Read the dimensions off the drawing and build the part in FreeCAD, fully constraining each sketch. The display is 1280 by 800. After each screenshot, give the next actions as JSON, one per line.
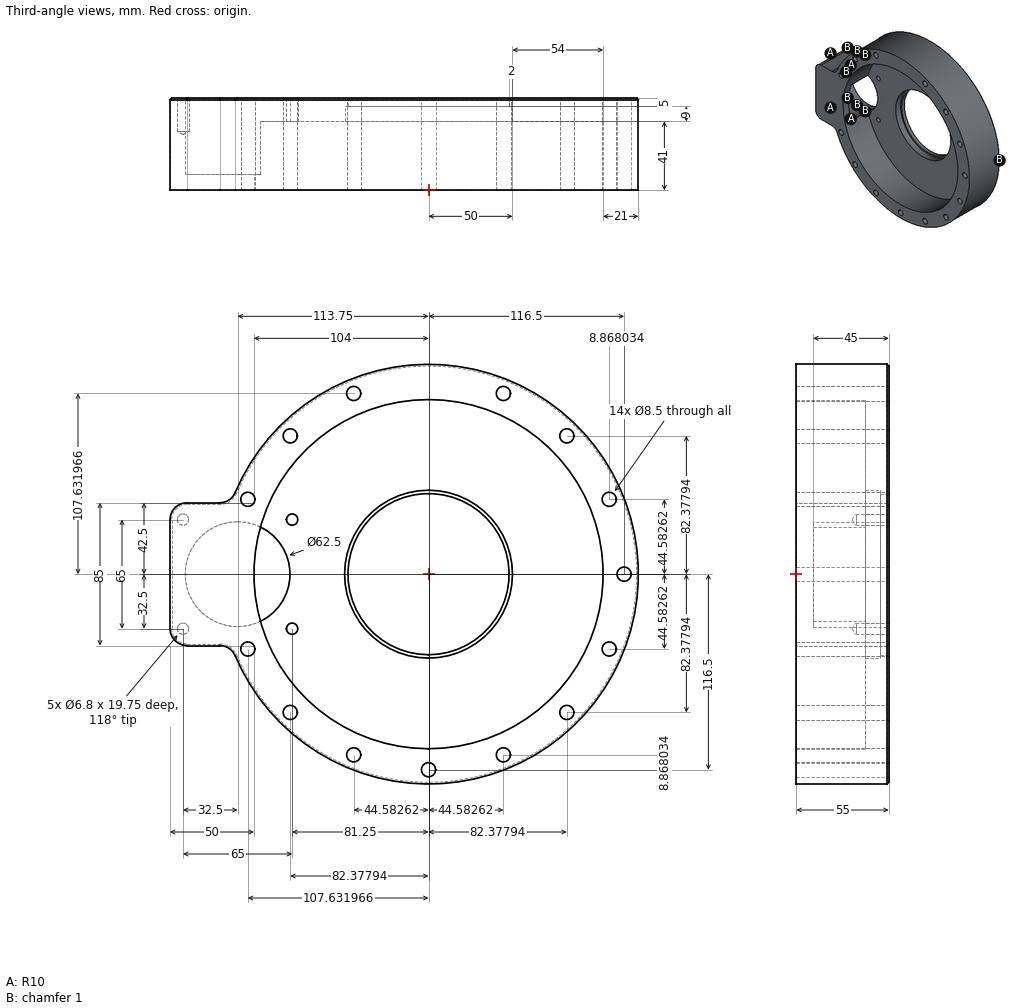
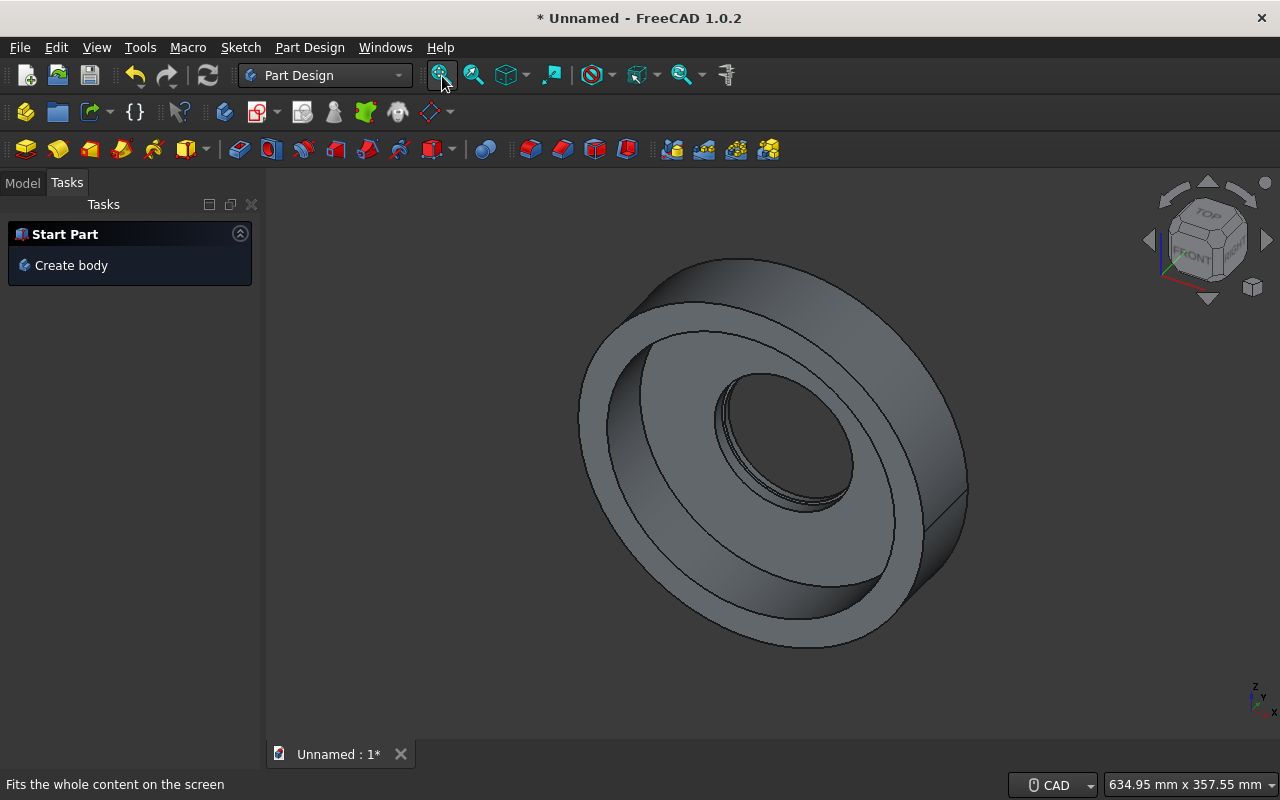
{"action": "key", "text": "4"}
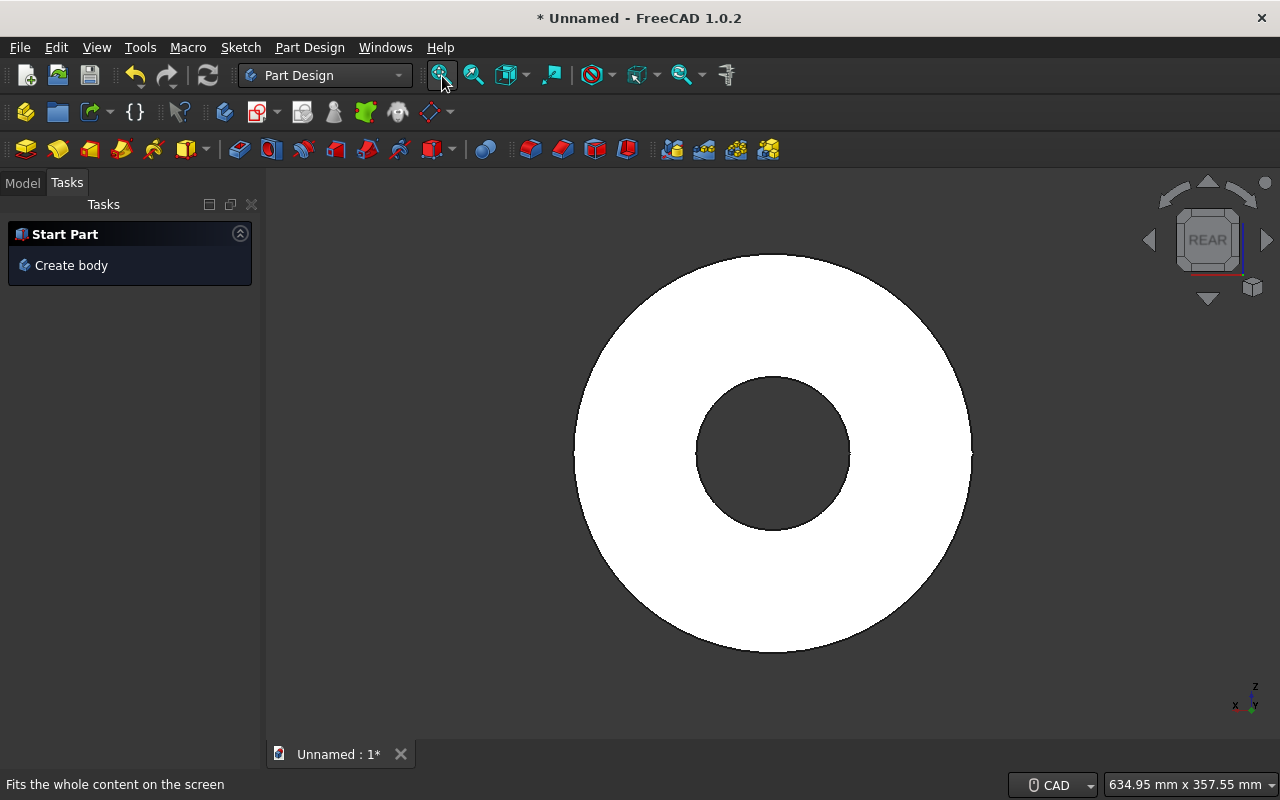
{"action": "left_click", "coordinate": [716, 567]}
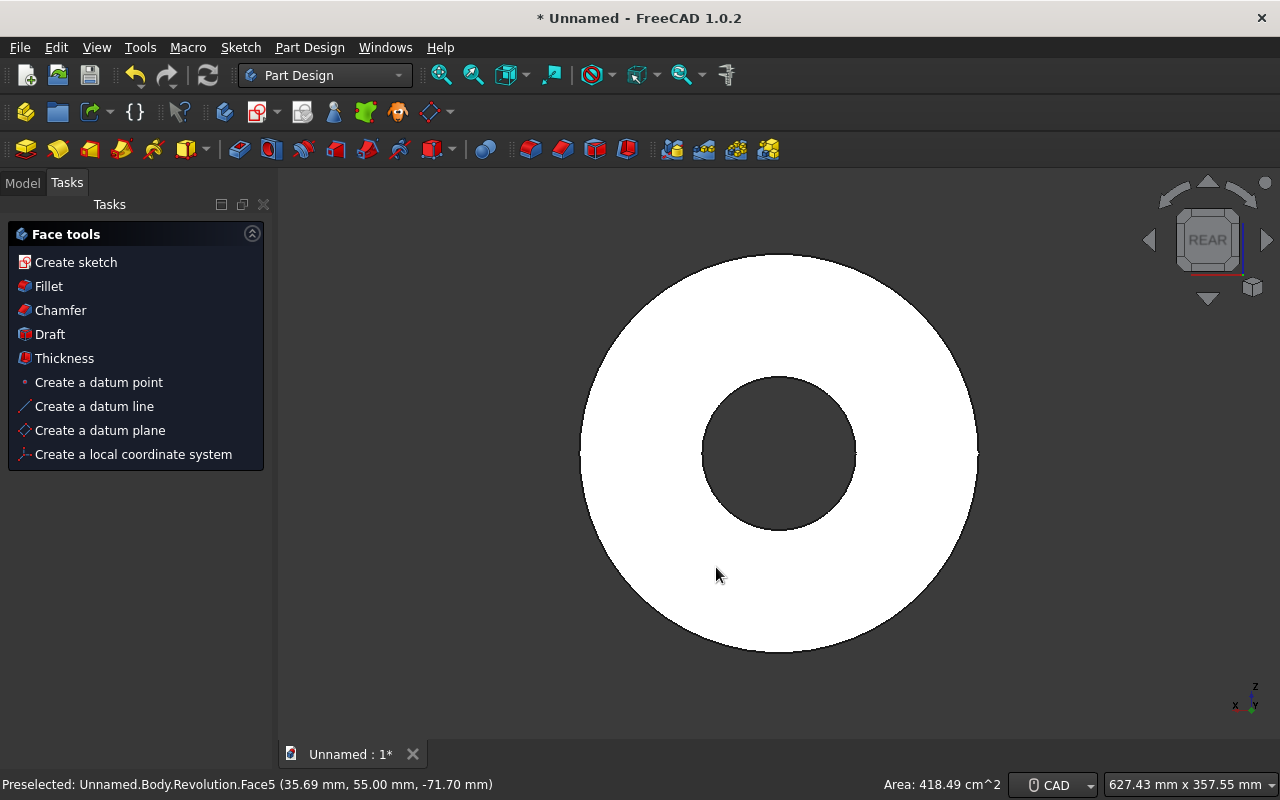
{"action": "left_click", "coordinate": [258, 112]}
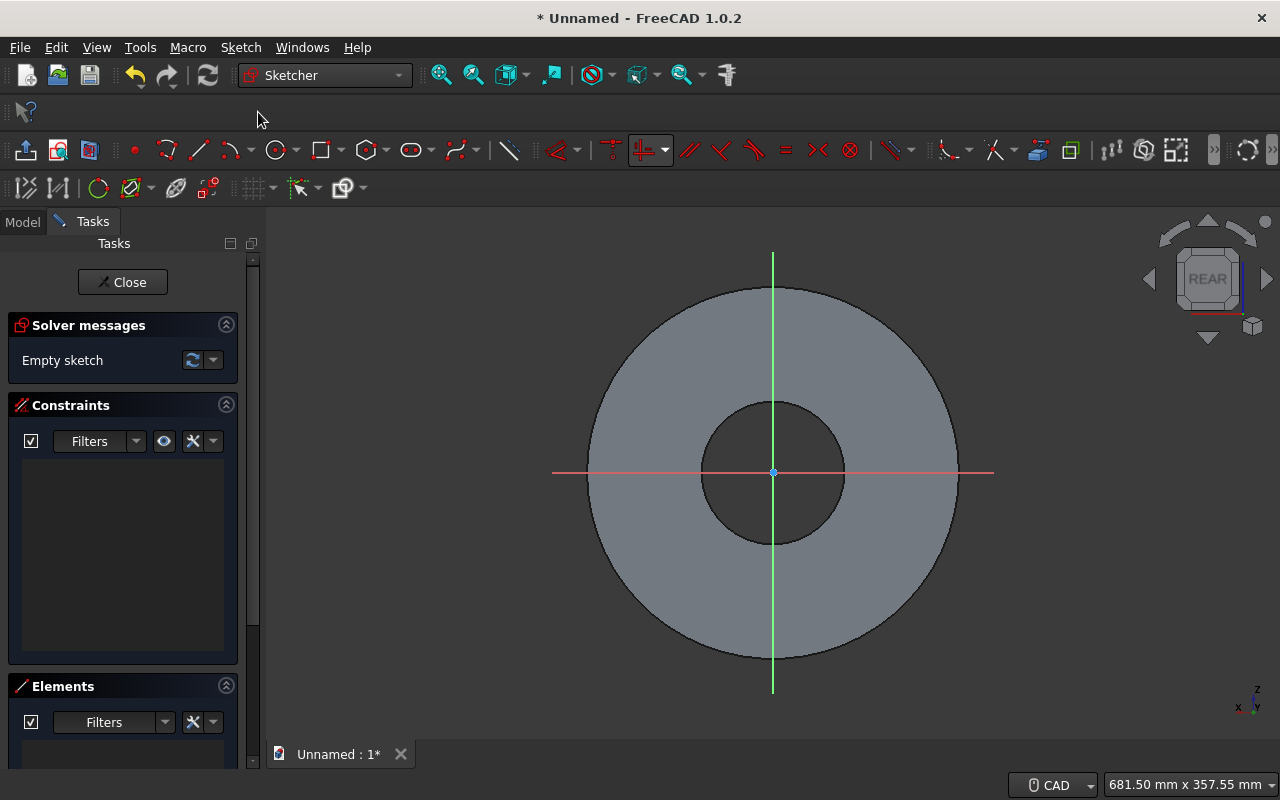
{"action": "scroll", "coordinate": [994, 473], "scroll_direction": "up", "scroll_amount": 5}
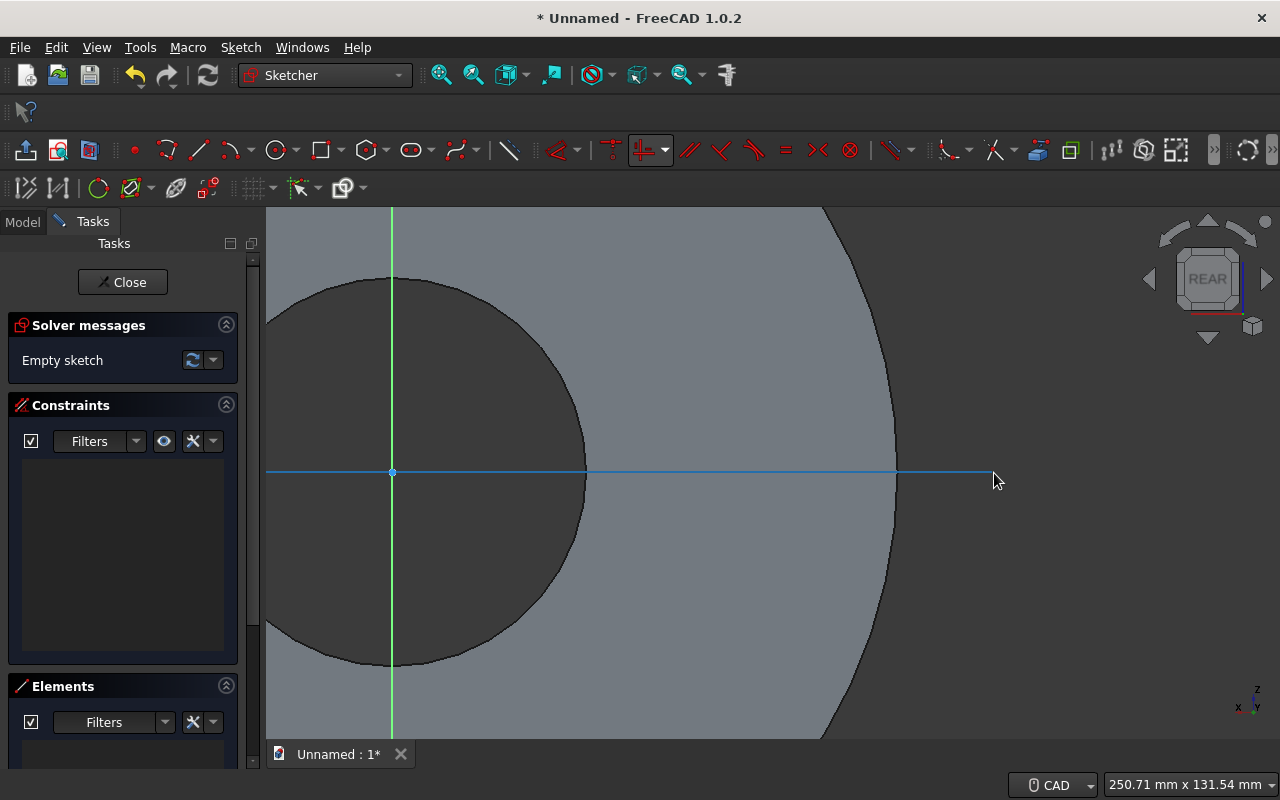
{"action": "key", "text": "g r"}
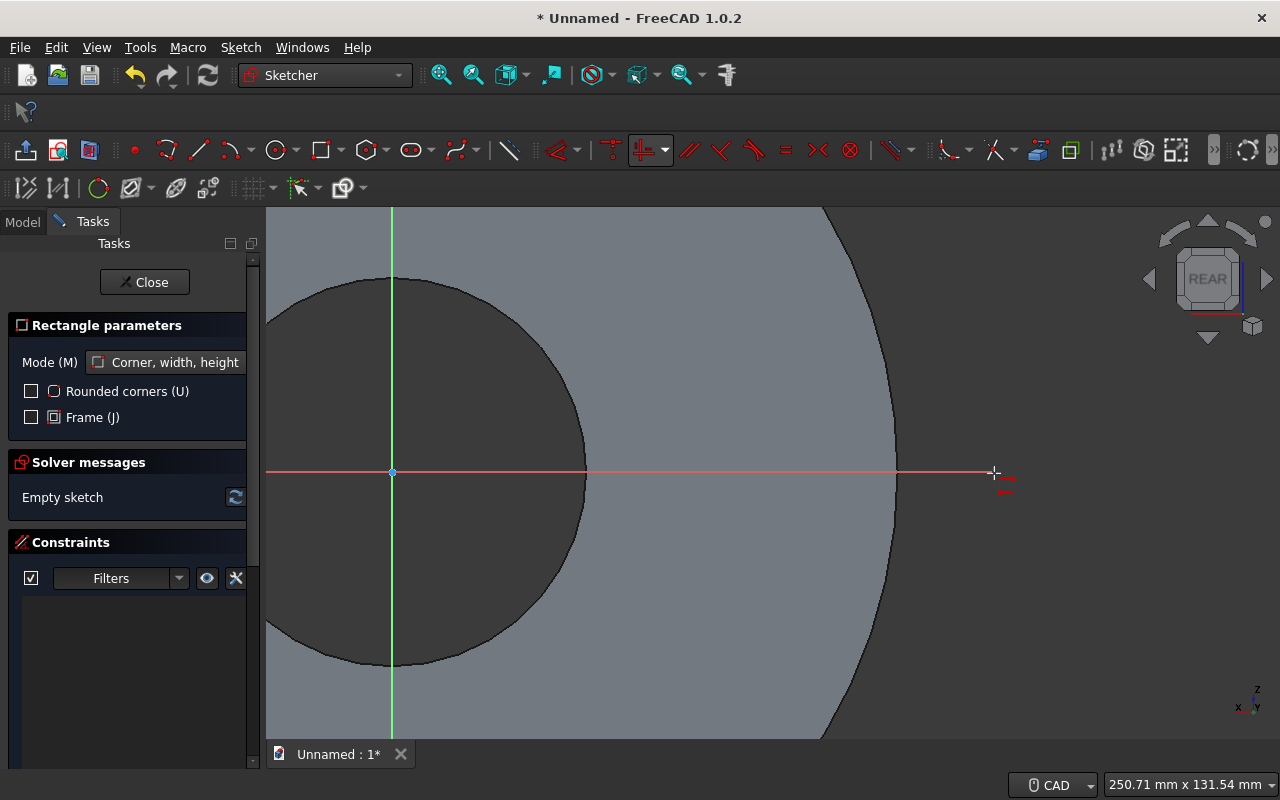
{"action": "left_click", "coordinate": [813, 300]}
{"action": "left_click", "coordinate": [1015, 644]}
{"action": "key", "text": "Escape"}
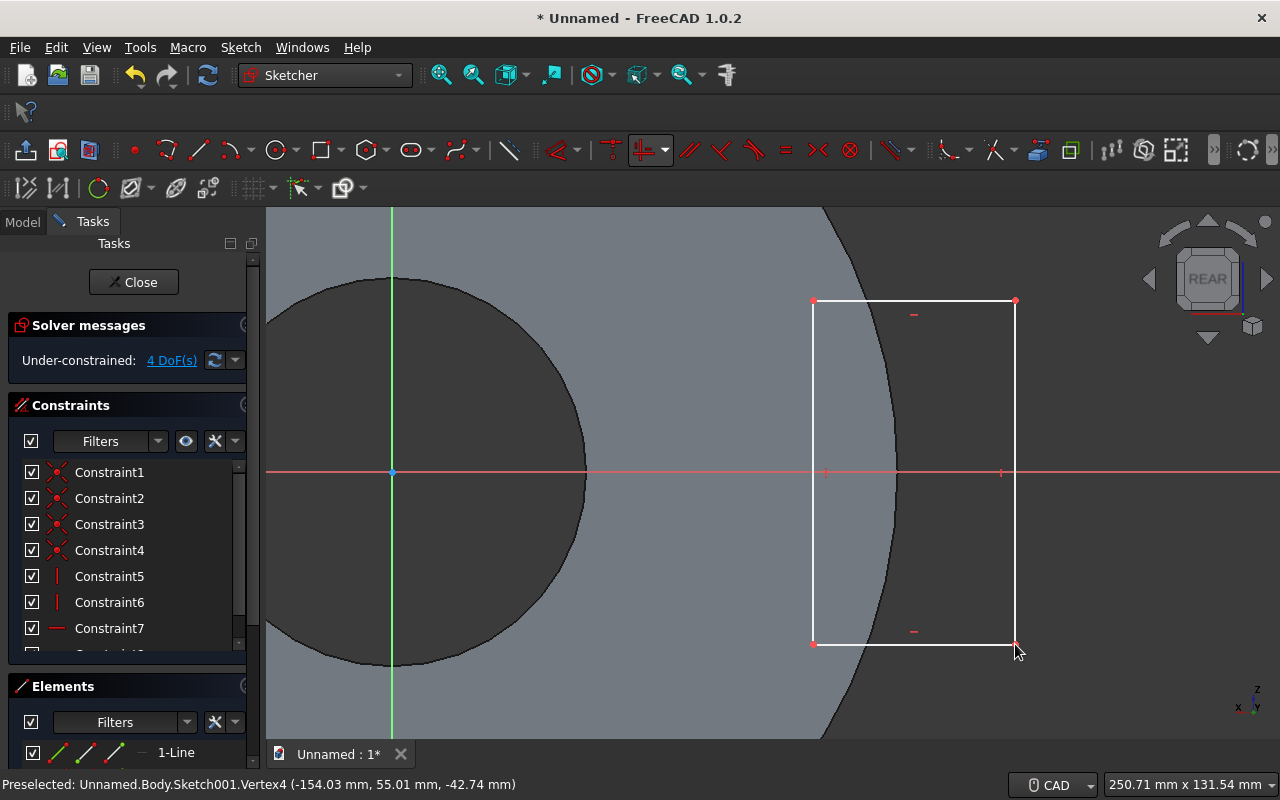
{"action": "left_click", "coordinate": [556, 150]}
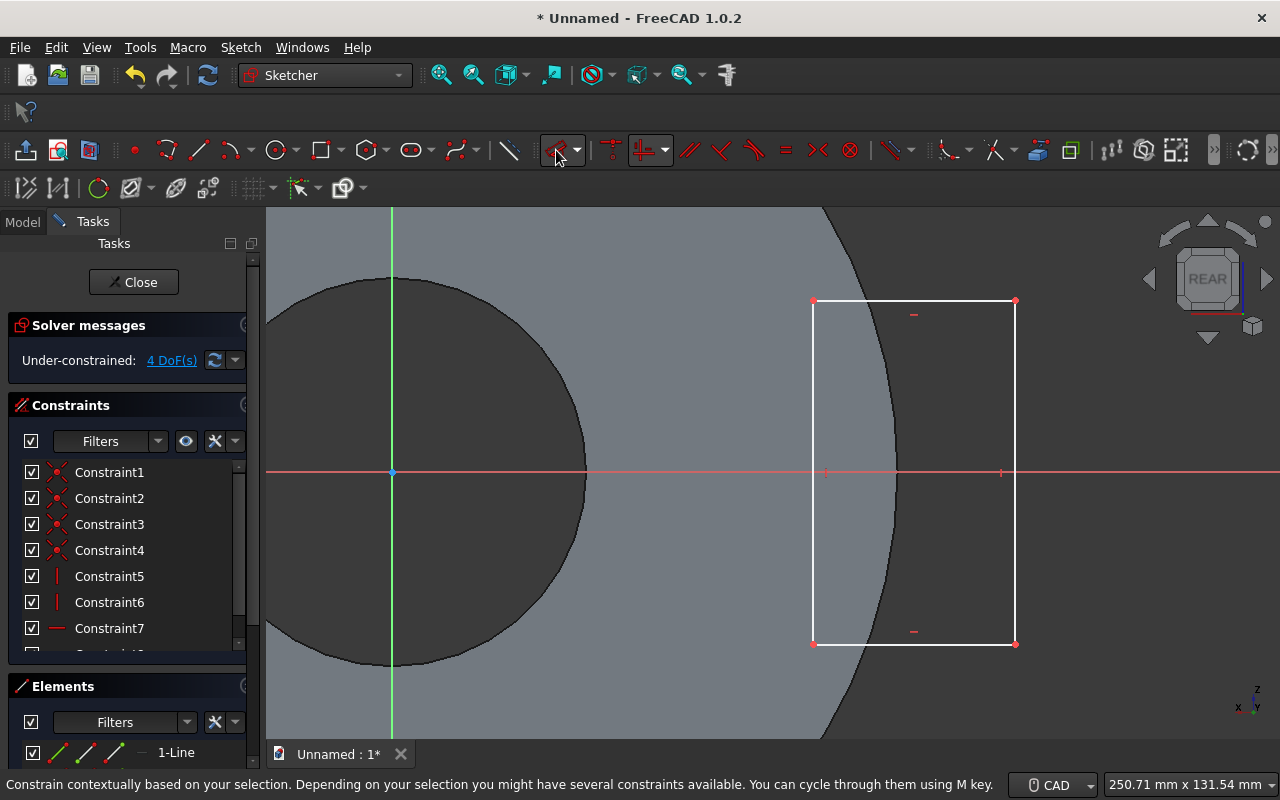
{"action": "left_click", "coordinate": [813, 404]}
{"action": "left_click", "coordinate": [847, 394]}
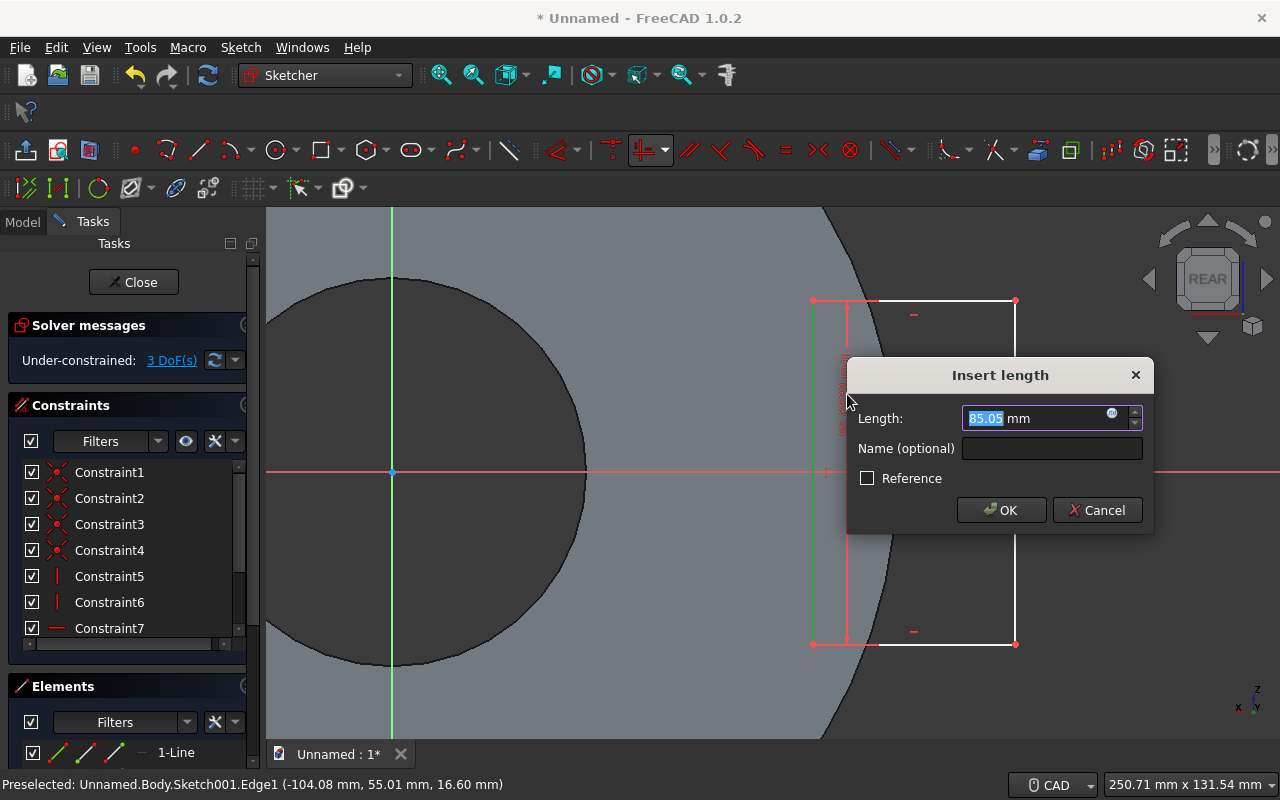
{"action": "type", "text": "85"}
{"action": "key", "text": "Return"}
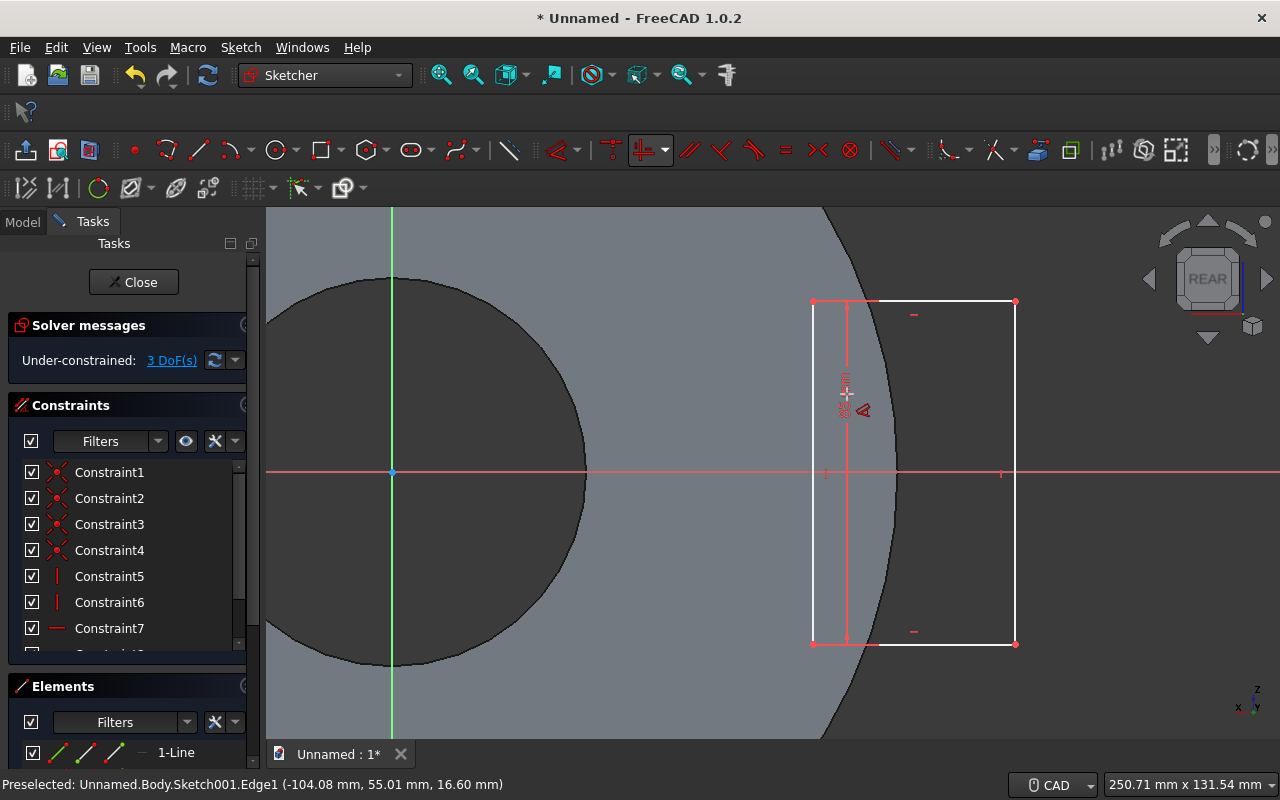
{"action": "left_click", "coordinate": [874, 645]}
{"action": "left_click", "coordinate": [914, 679]}